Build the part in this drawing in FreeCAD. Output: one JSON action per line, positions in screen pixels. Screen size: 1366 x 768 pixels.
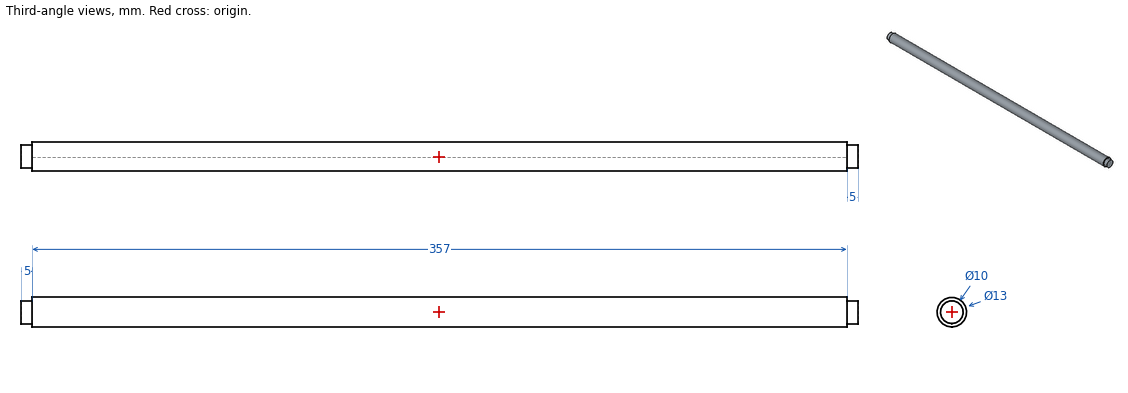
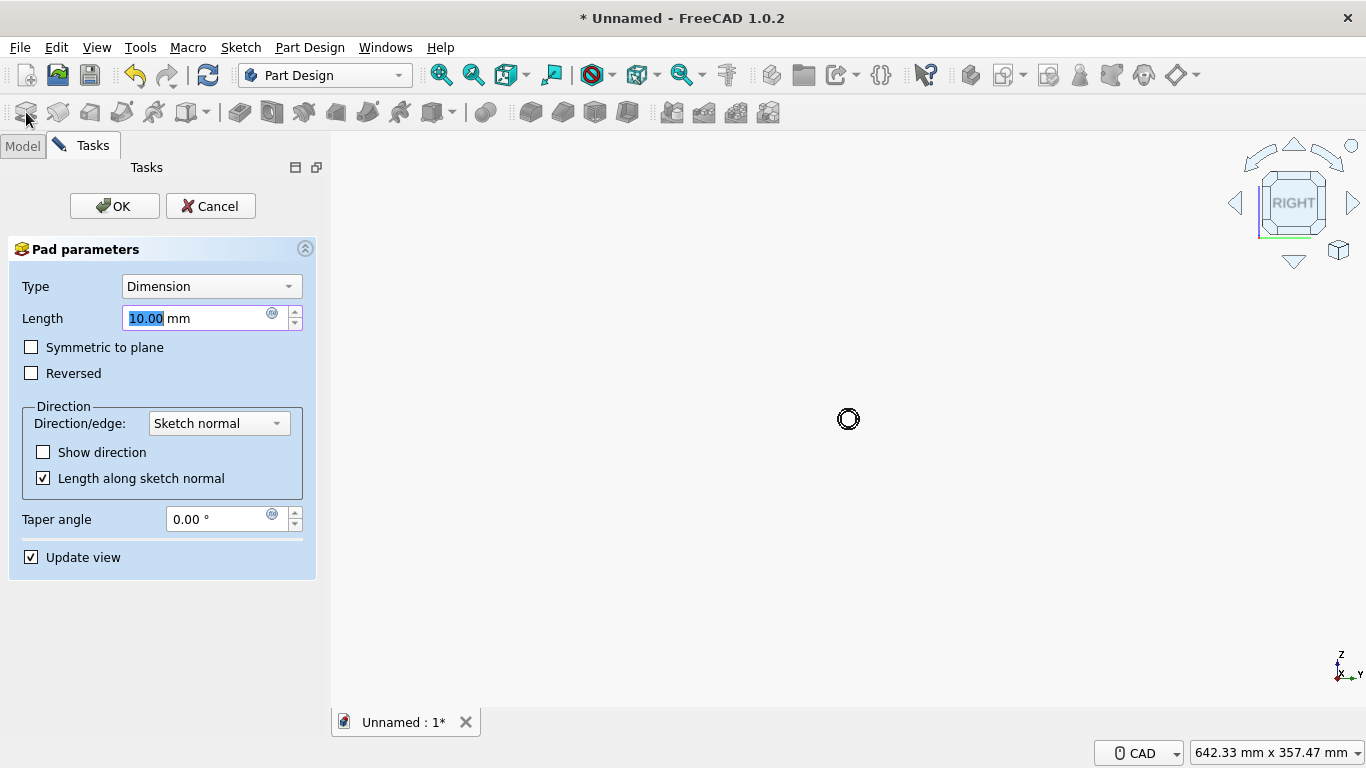
{"action": "type", "text": "5"}
{"action": "key", "text": "Tab"}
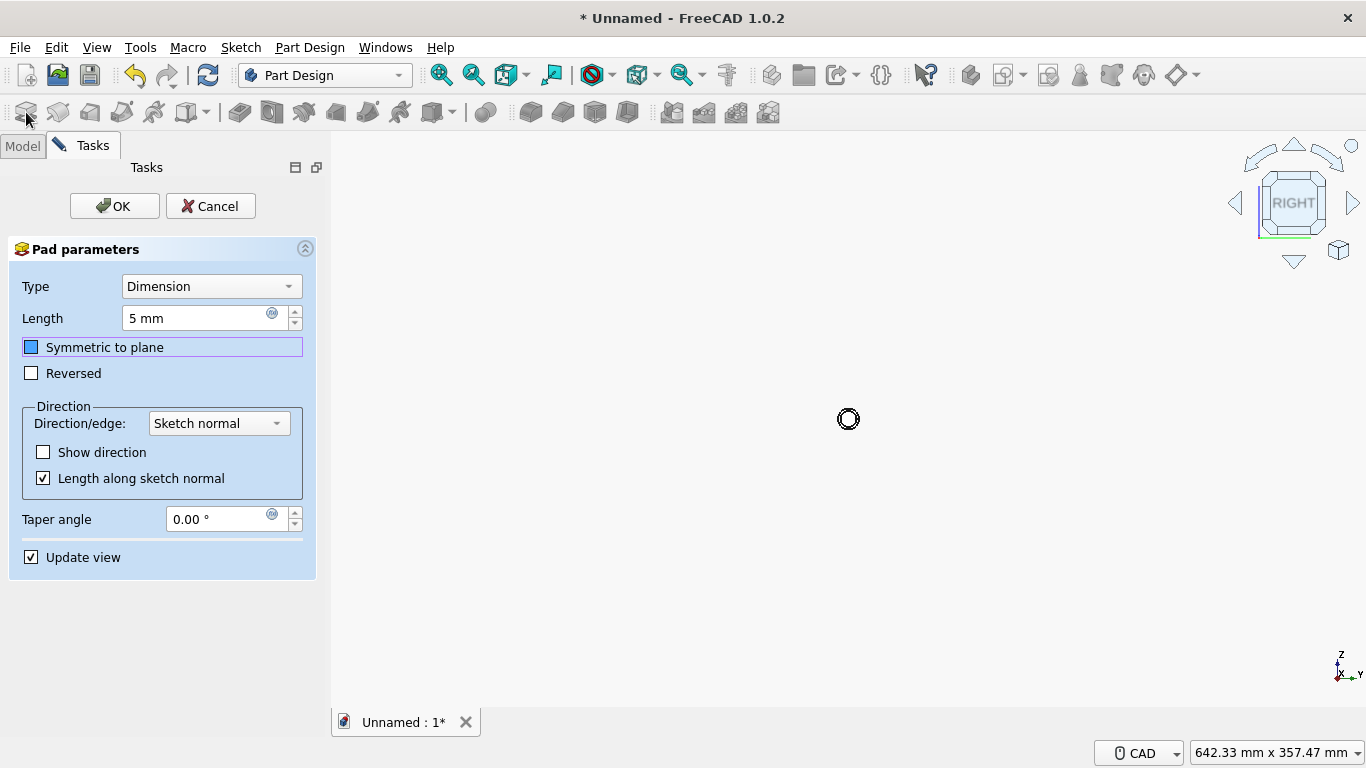
{"action": "left_click", "coordinate": [115, 206]}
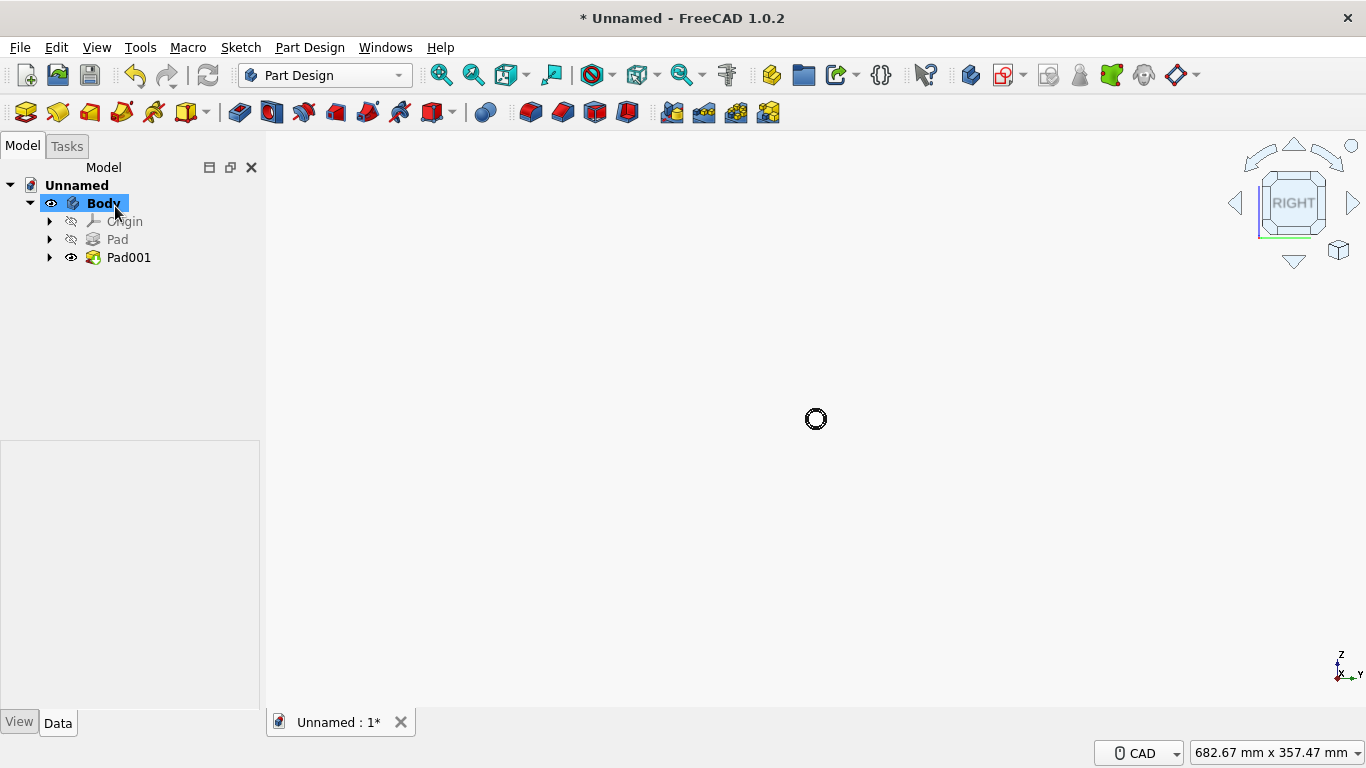
{"action": "left_click", "coordinate": [442, 76]}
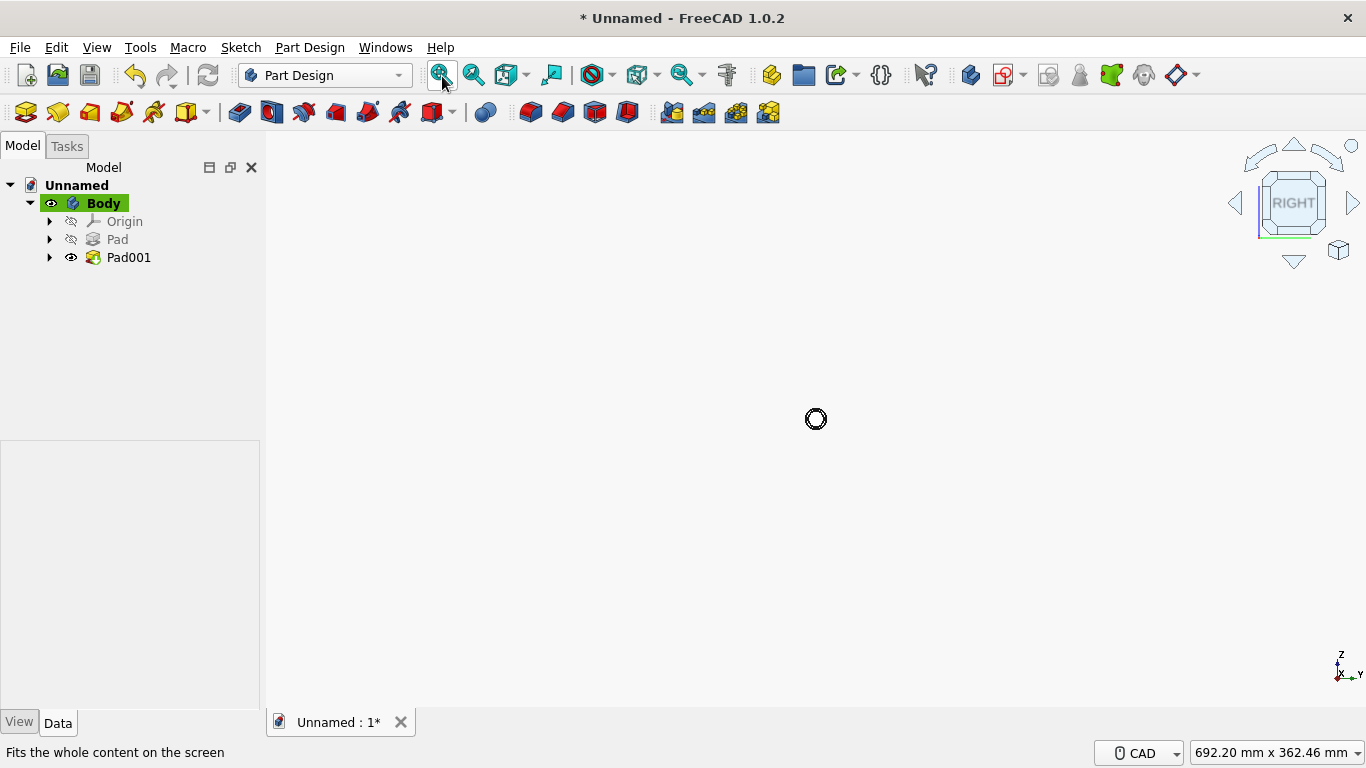
{"action": "left_click", "coordinate": [50, 221]}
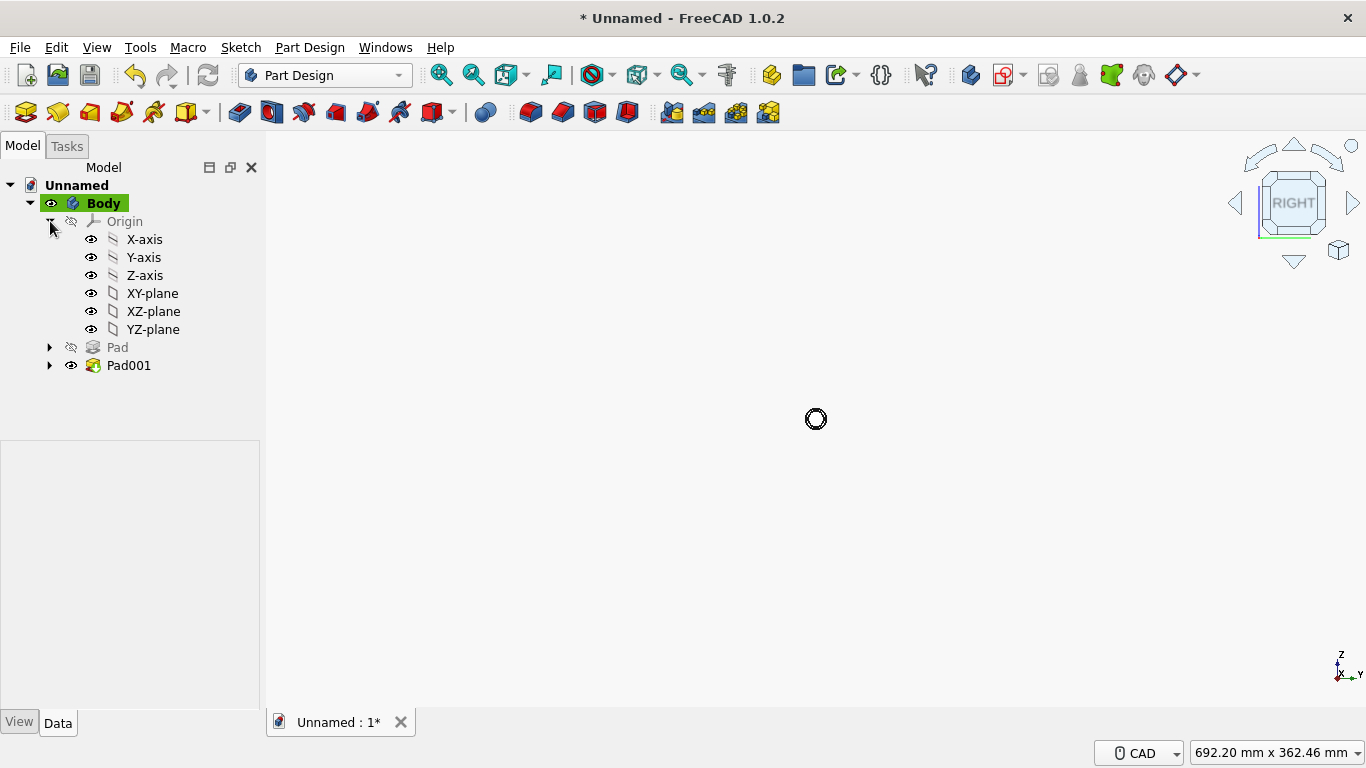
{"action": "left_click", "coordinate": [136, 329]}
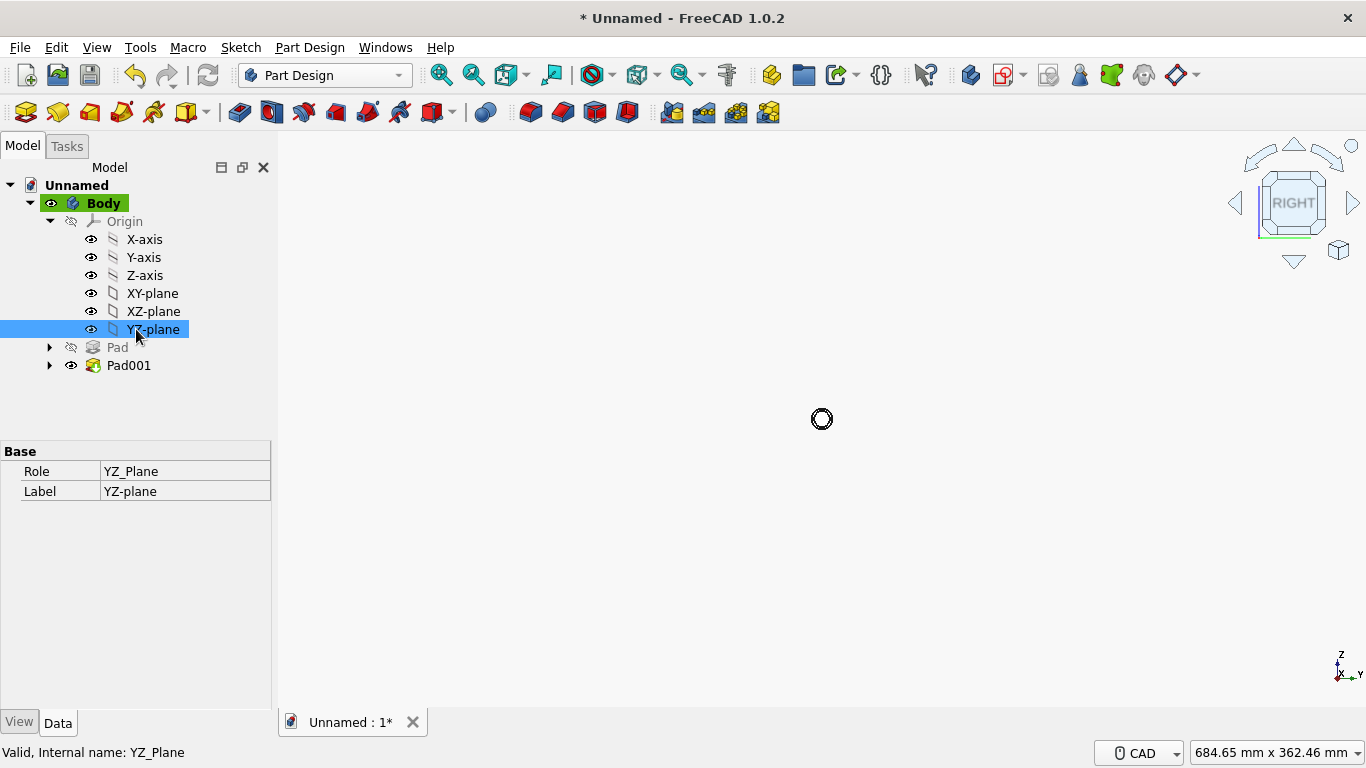
{"action": "left_click", "coordinate": [1176, 76]}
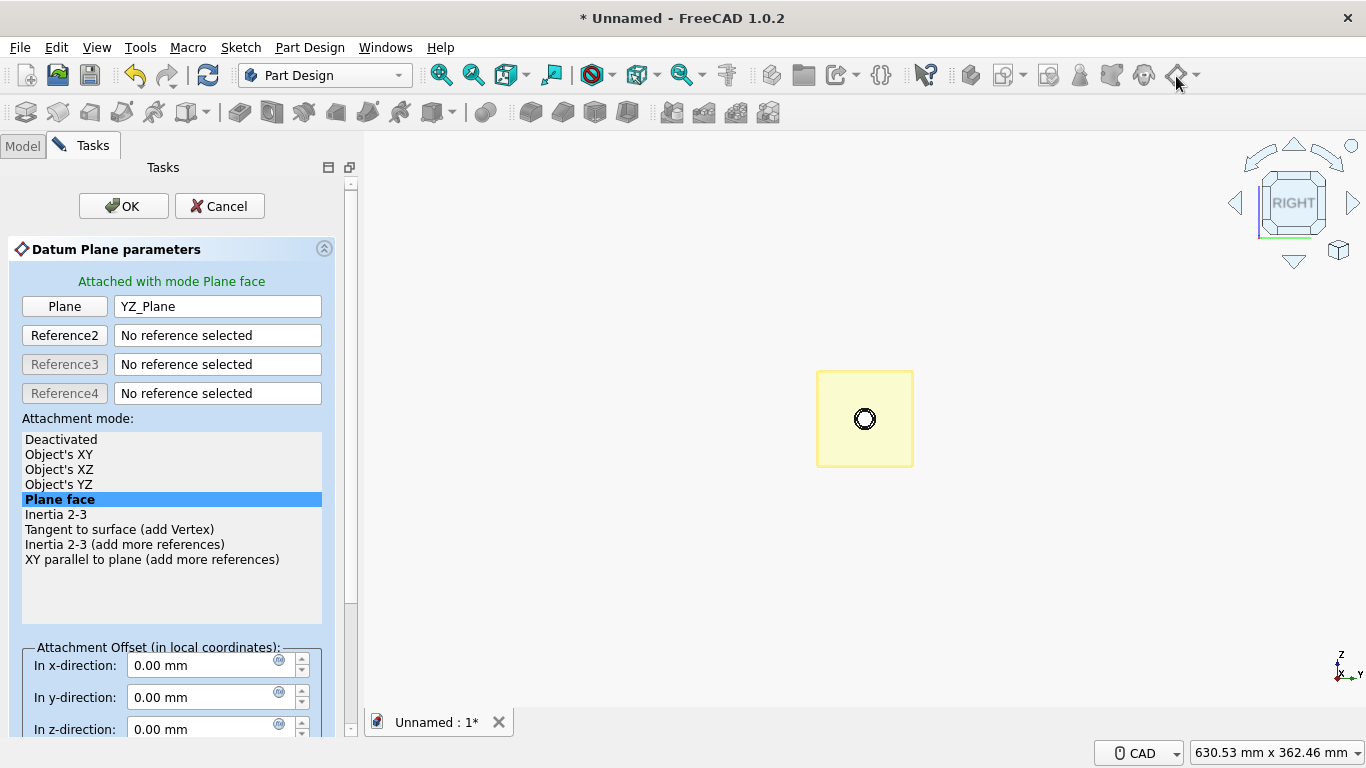
{"action": "scroll", "coordinate": [351, 456], "scroll_direction": "down", "scroll_amount": 2}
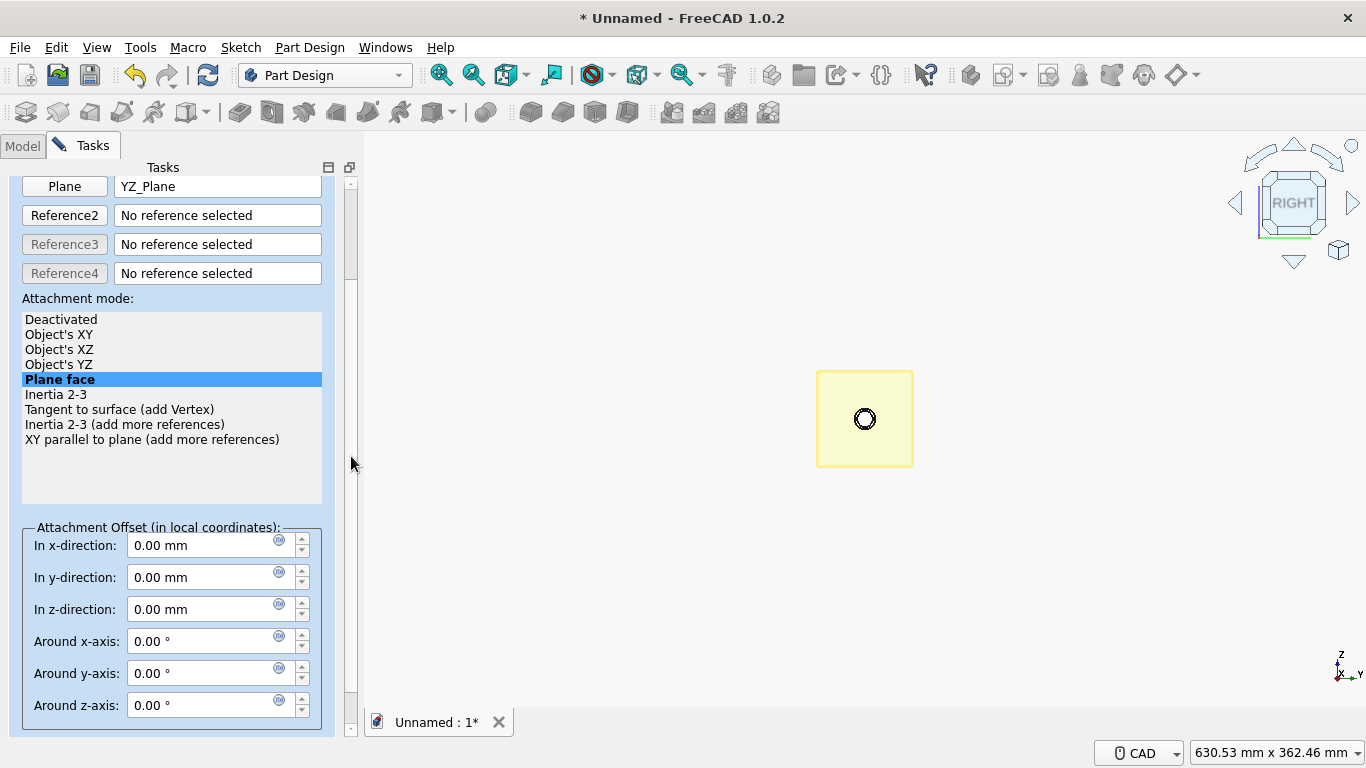
{"action": "triple_click", "coordinate": [210, 609]}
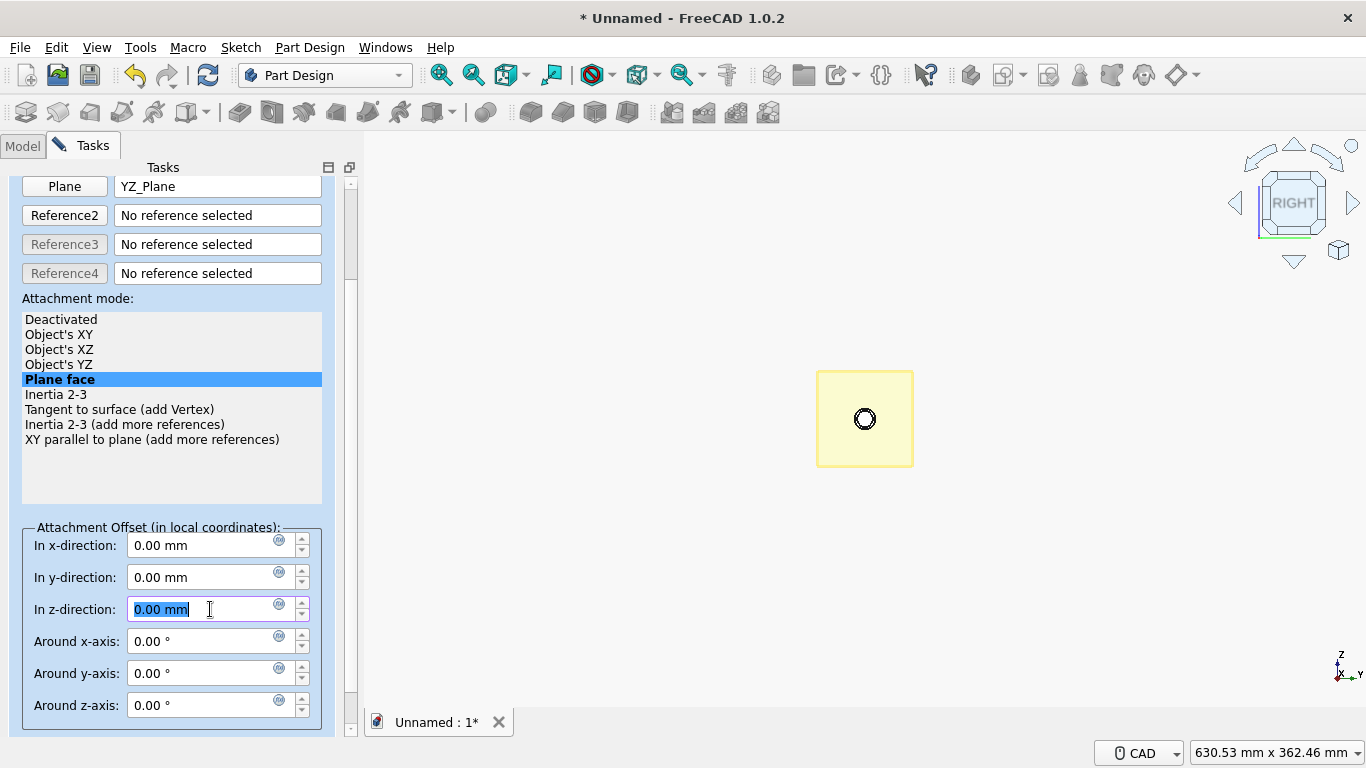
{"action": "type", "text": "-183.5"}
{"action": "key", "text": "Tab"}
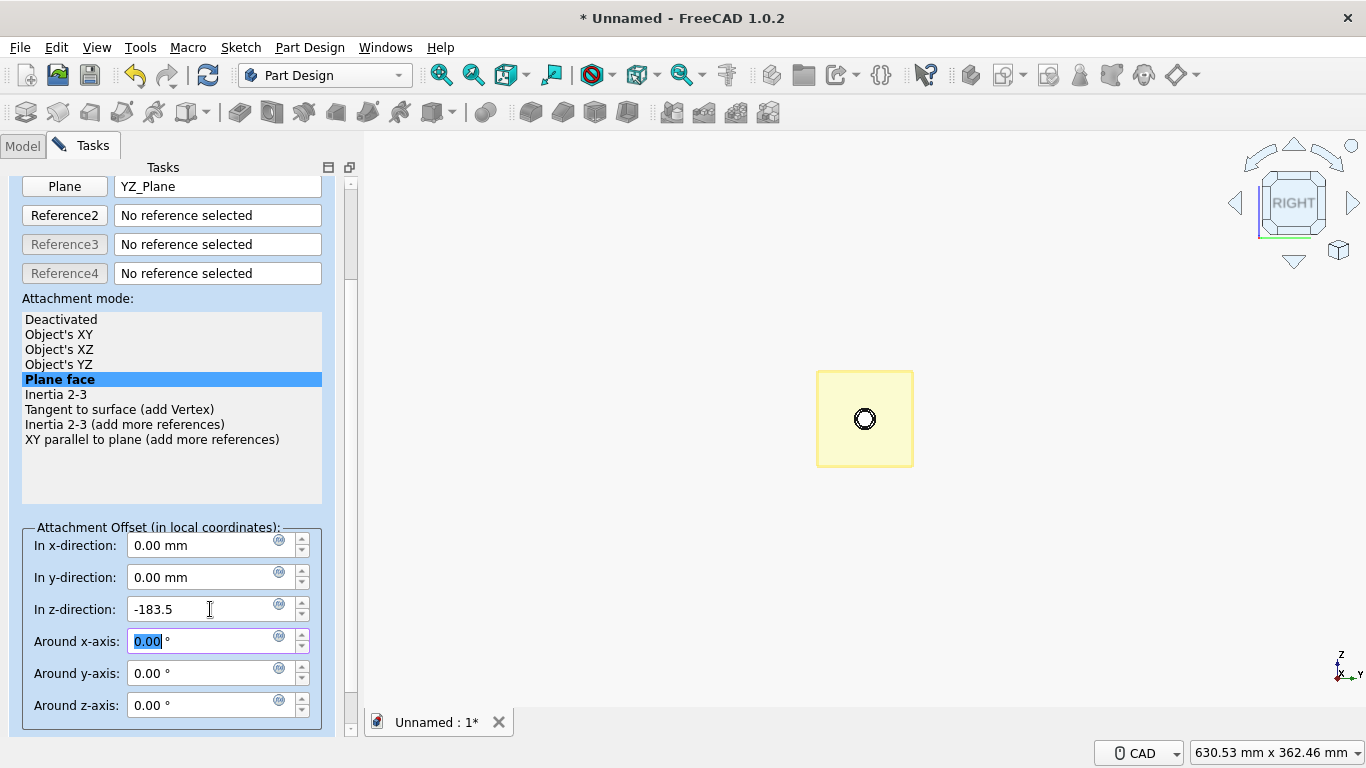
{"action": "scroll", "coordinate": [351, 456], "scroll_direction": "up", "scroll_amount": 3}